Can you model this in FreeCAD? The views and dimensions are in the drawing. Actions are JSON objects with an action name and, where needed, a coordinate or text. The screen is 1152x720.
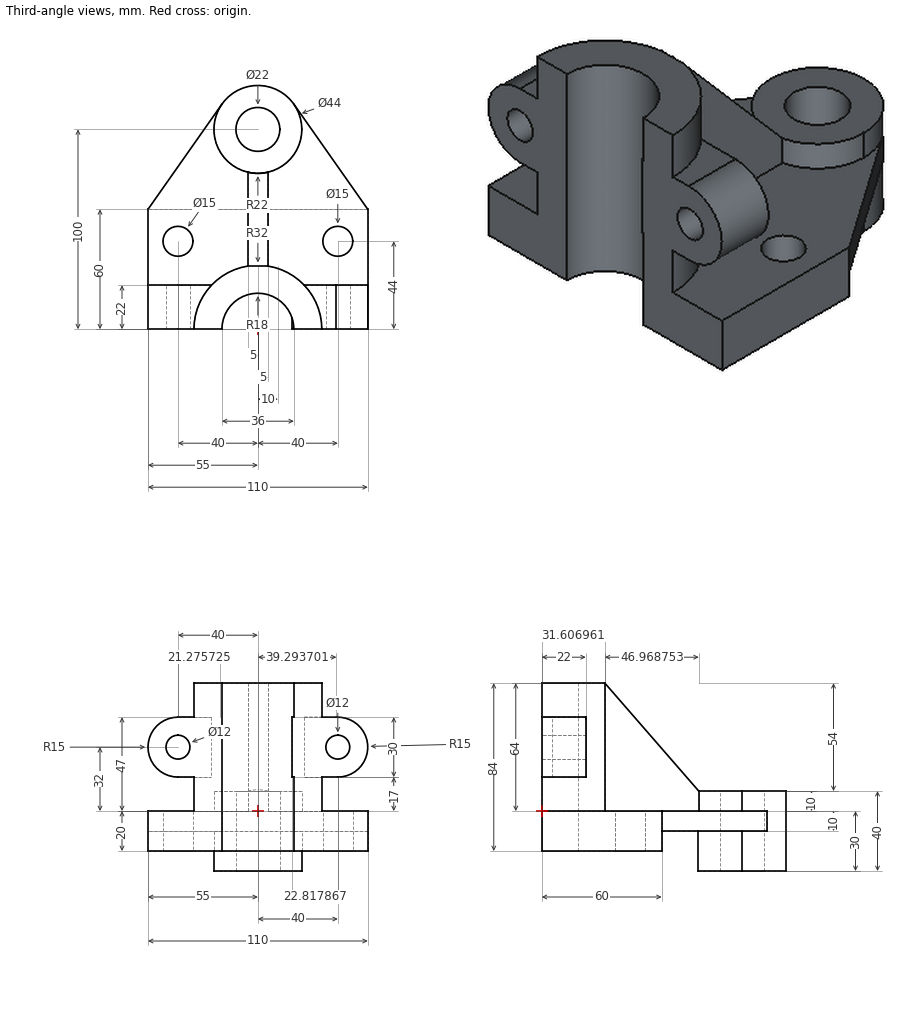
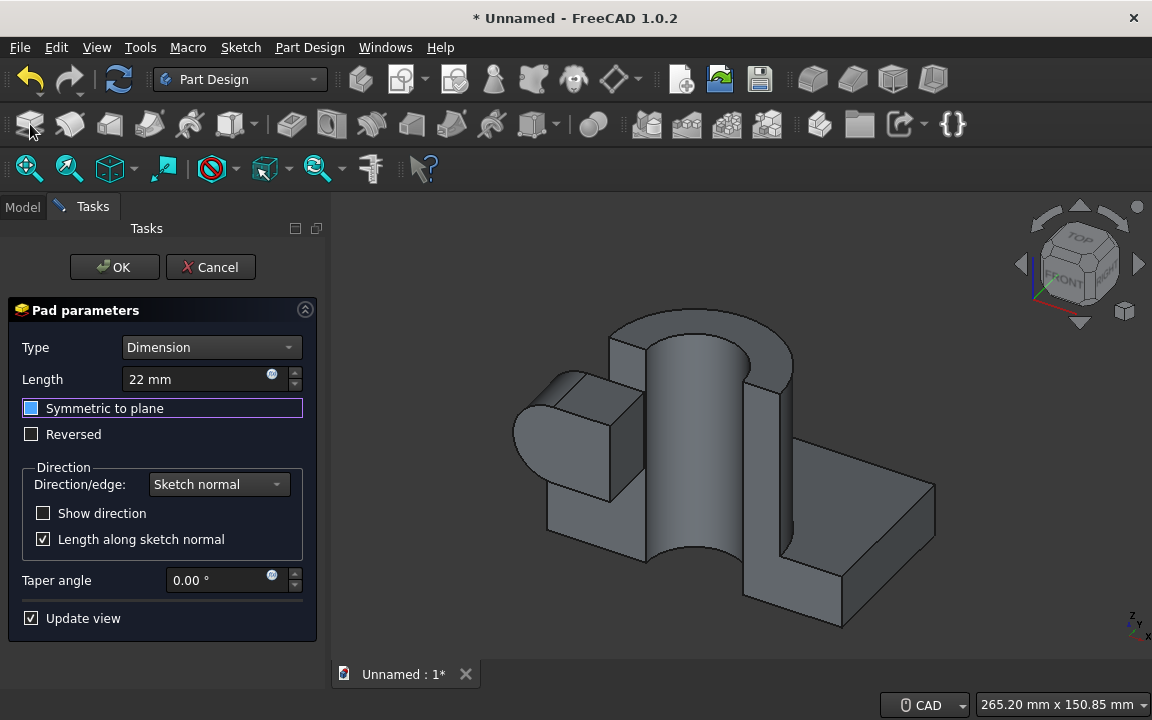
{"action": "left_click", "coordinate": [30, 434]}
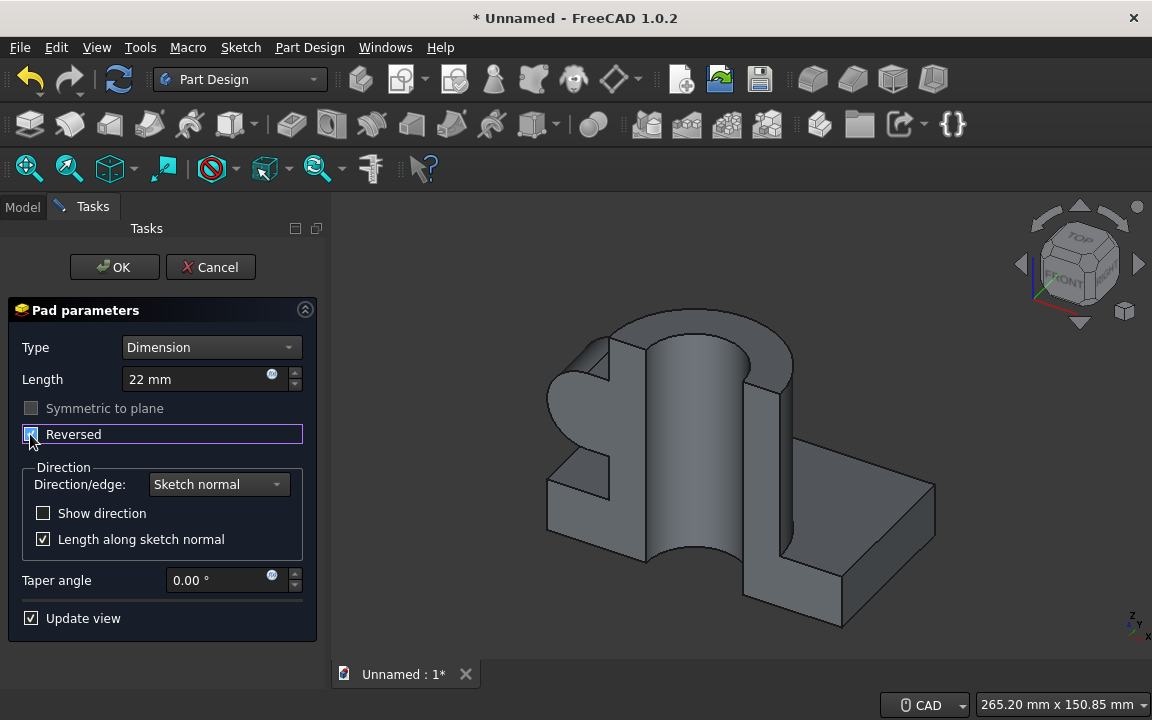
{"action": "left_click", "coordinate": [115, 267]}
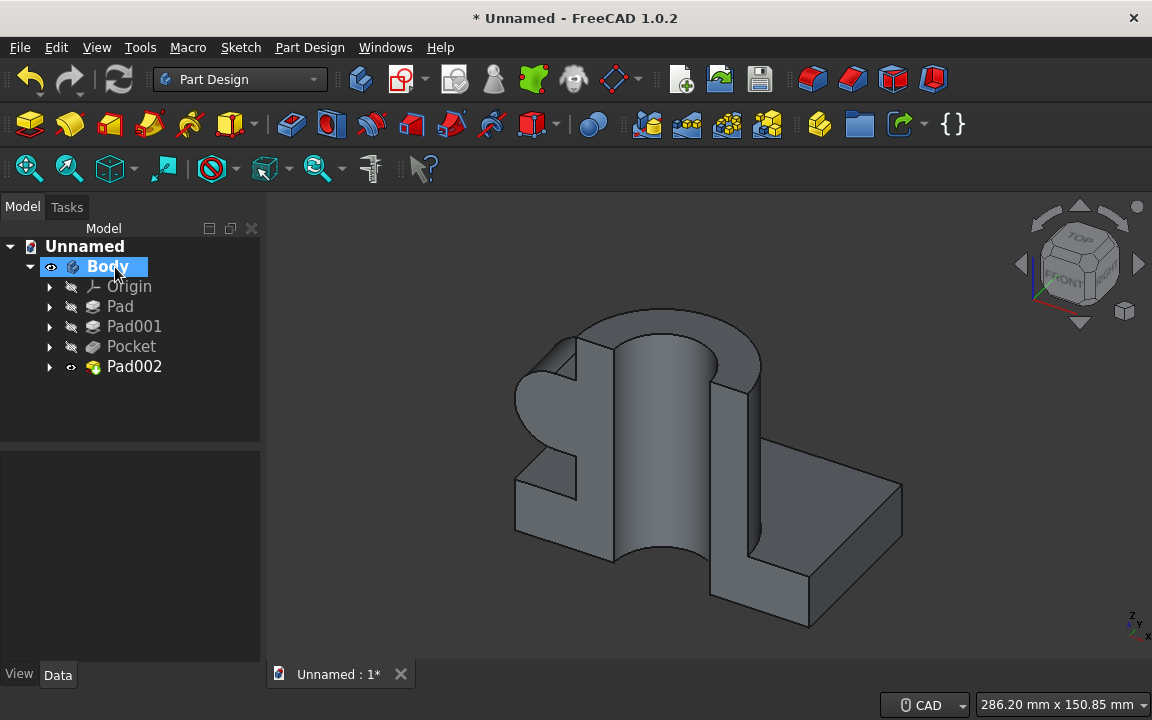
{"action": "key", "text": "4"}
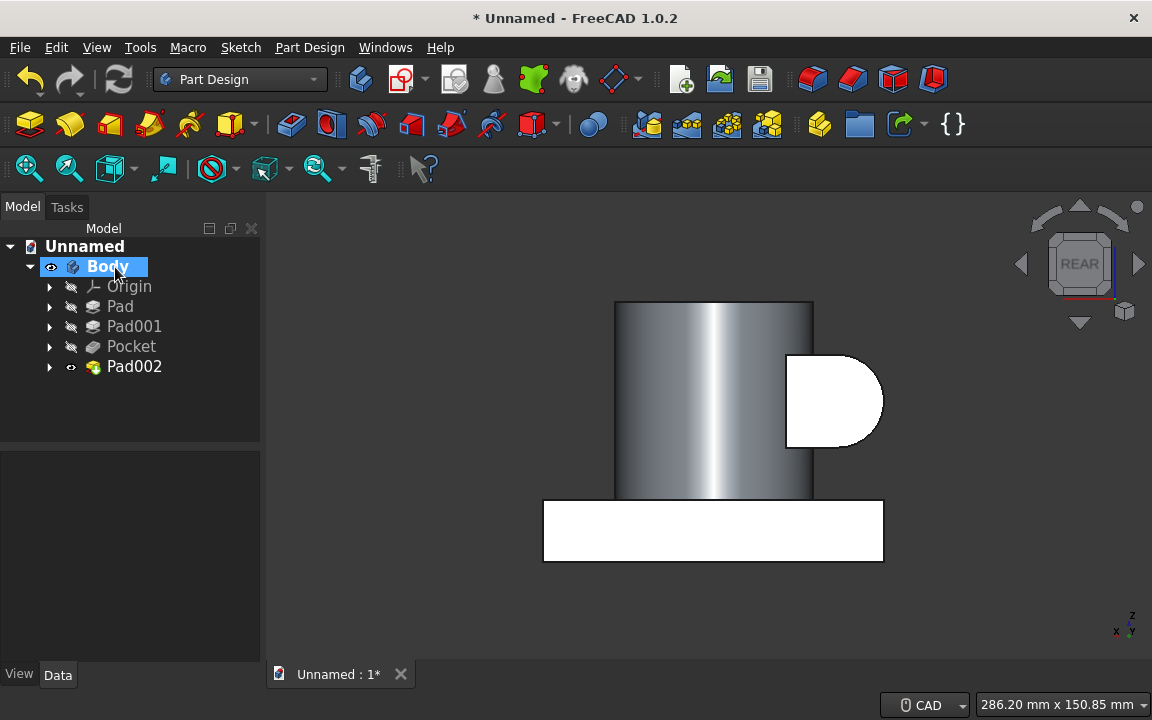
{"action": "left_click", "coordinate": [835, 400]}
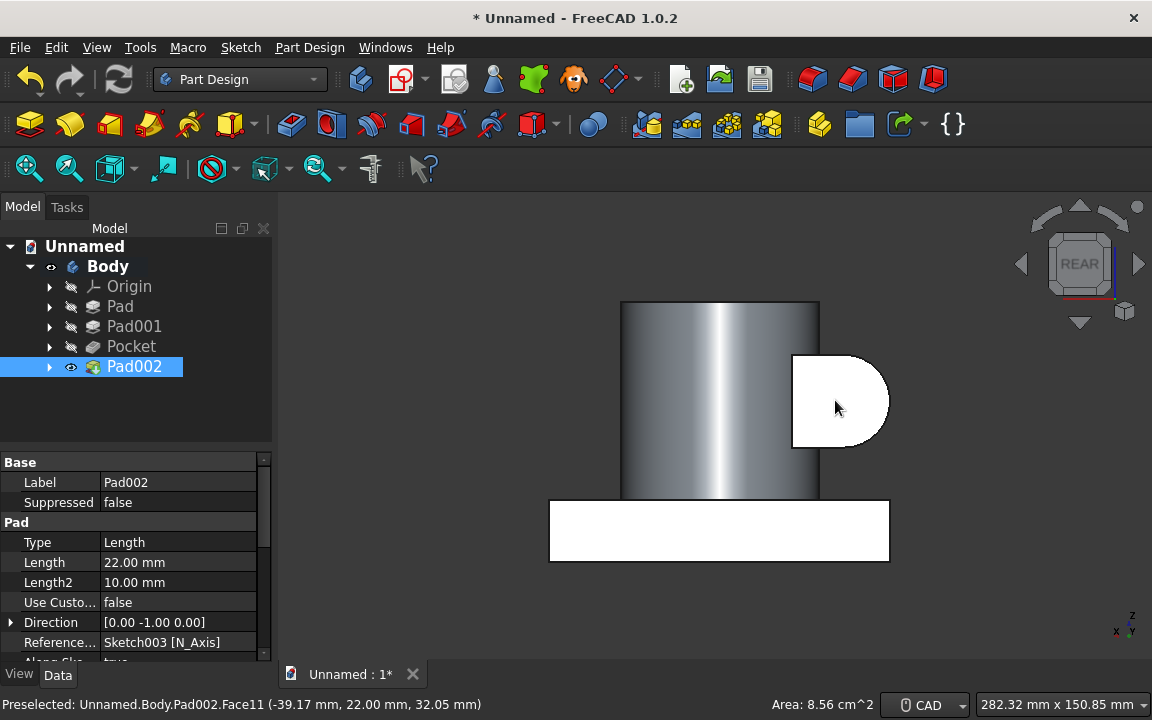
{"action": "left_click", "coordinate": [402, 80]}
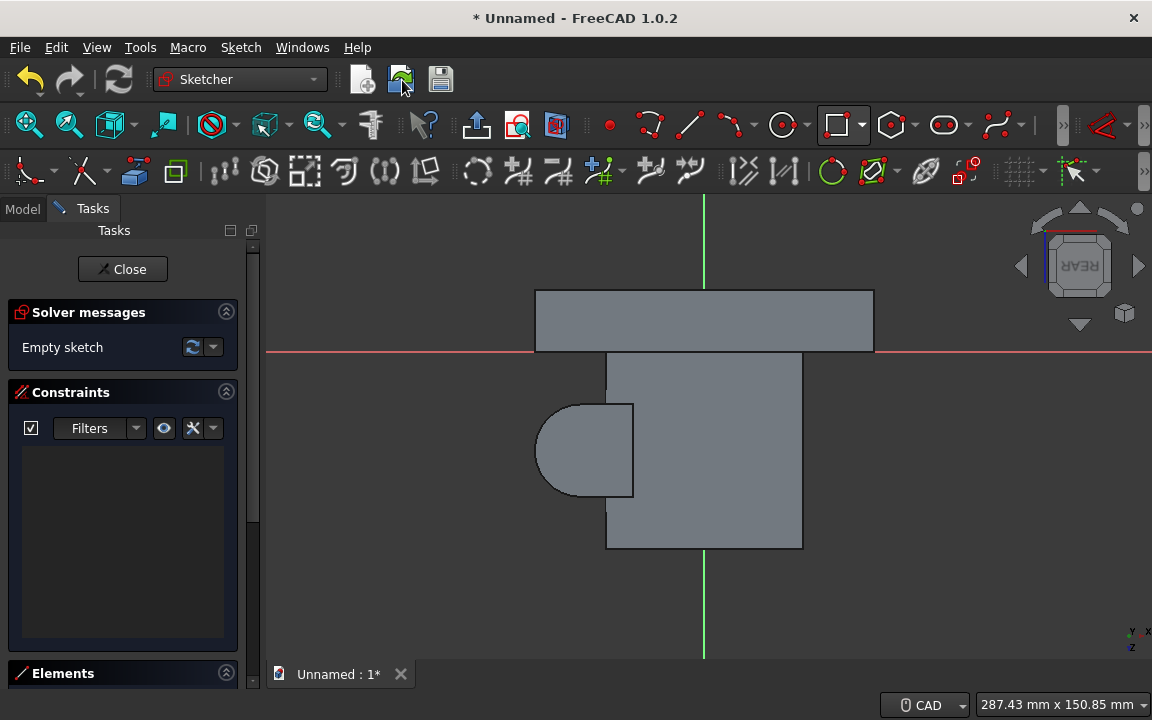
{"action": "left_click", "coordinate": [558, 126]}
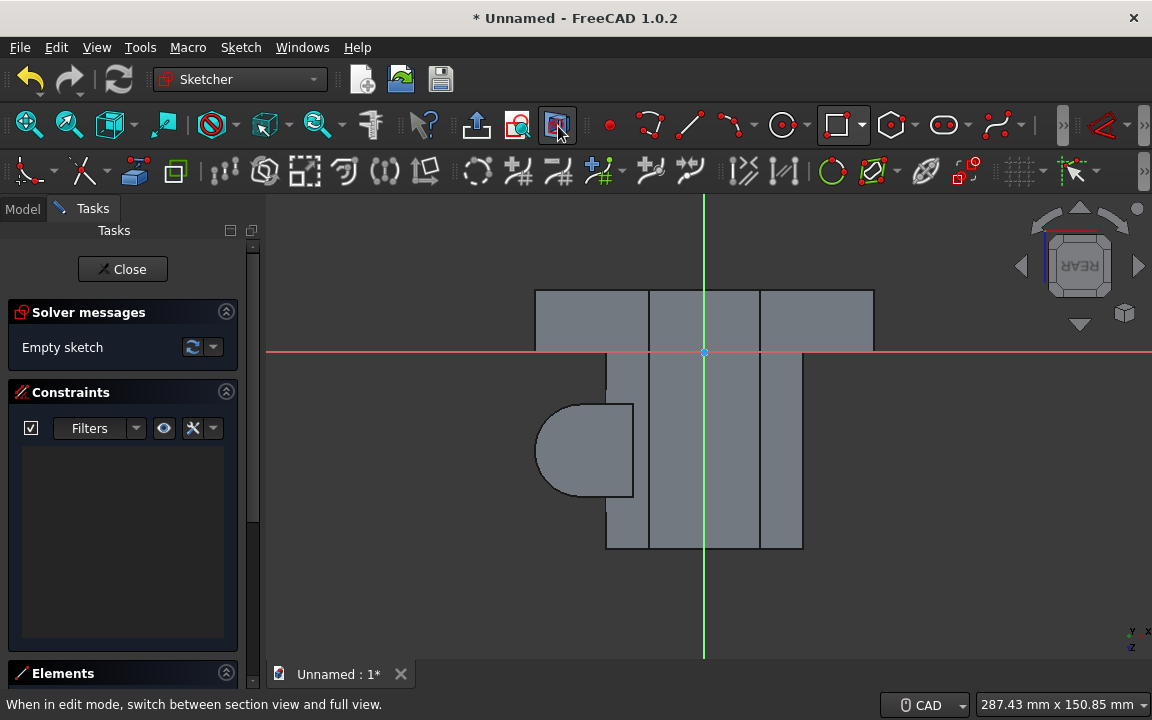
{"action": "scroll", "coordinate": [572, 455], "scroll_direction": "up", "scroll_amount": 10}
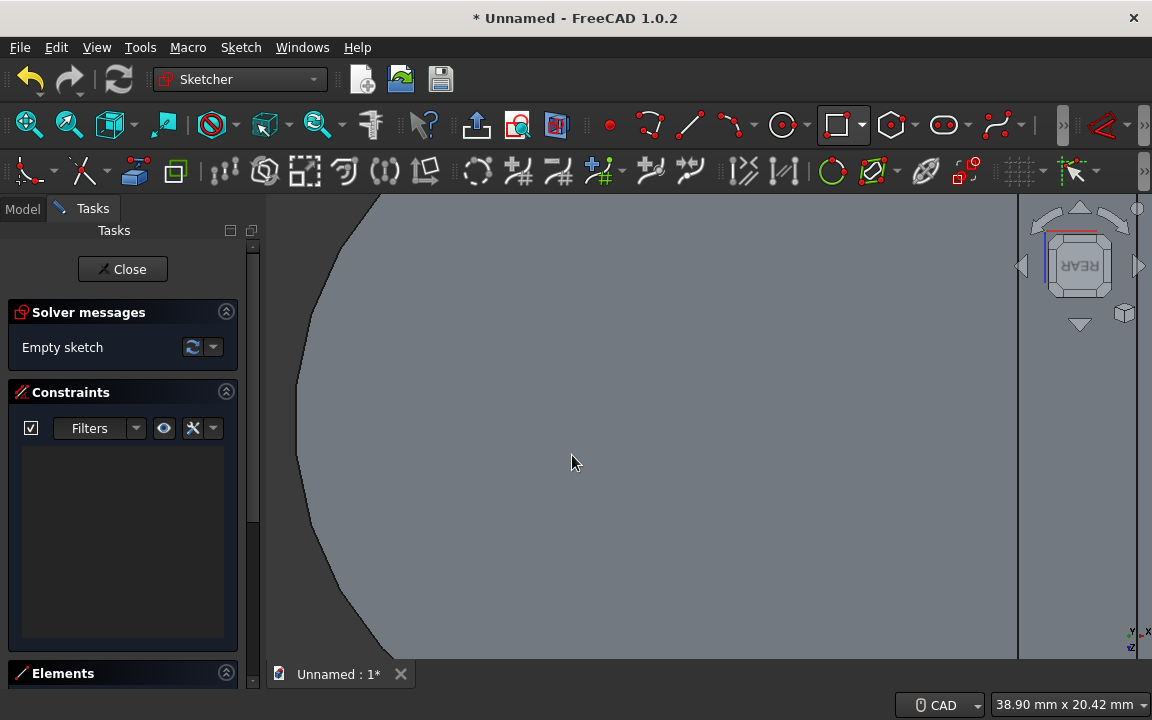
{"action": "left_click", "coordinate": [784, 126]}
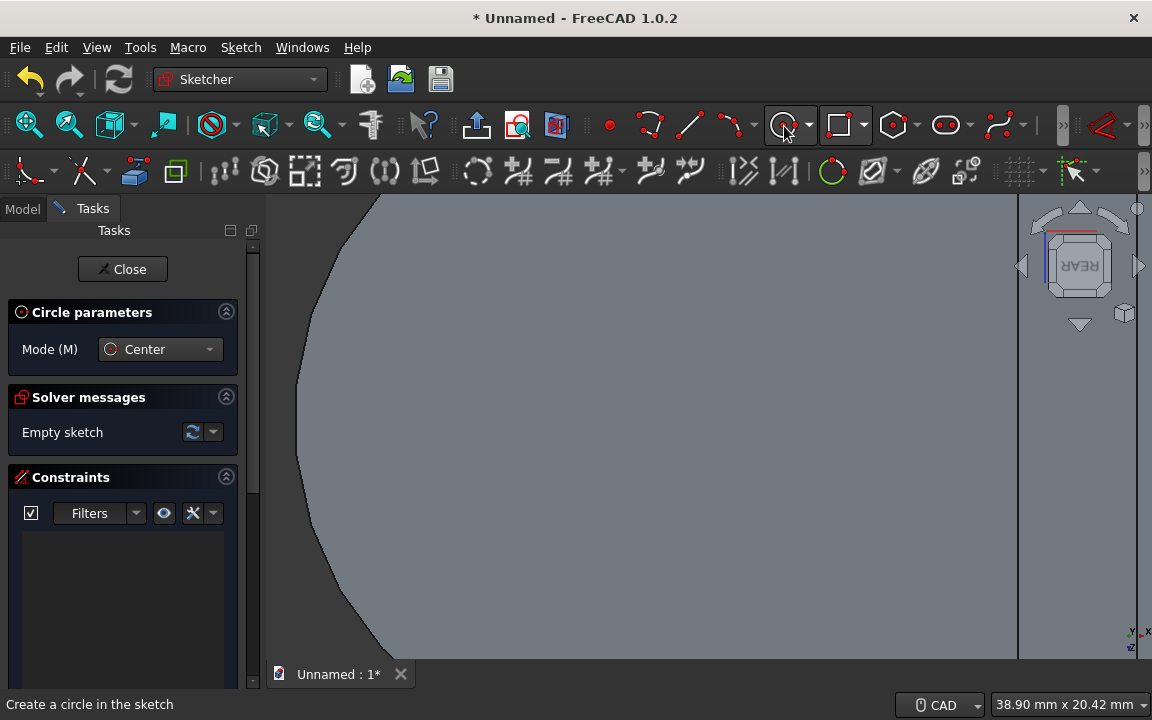
{"action": "left_click", "coordinate": [636, 420]}
{"action": "left_click", "coordinate": [733, 323]}
{"action": "key", "text": "Escape"}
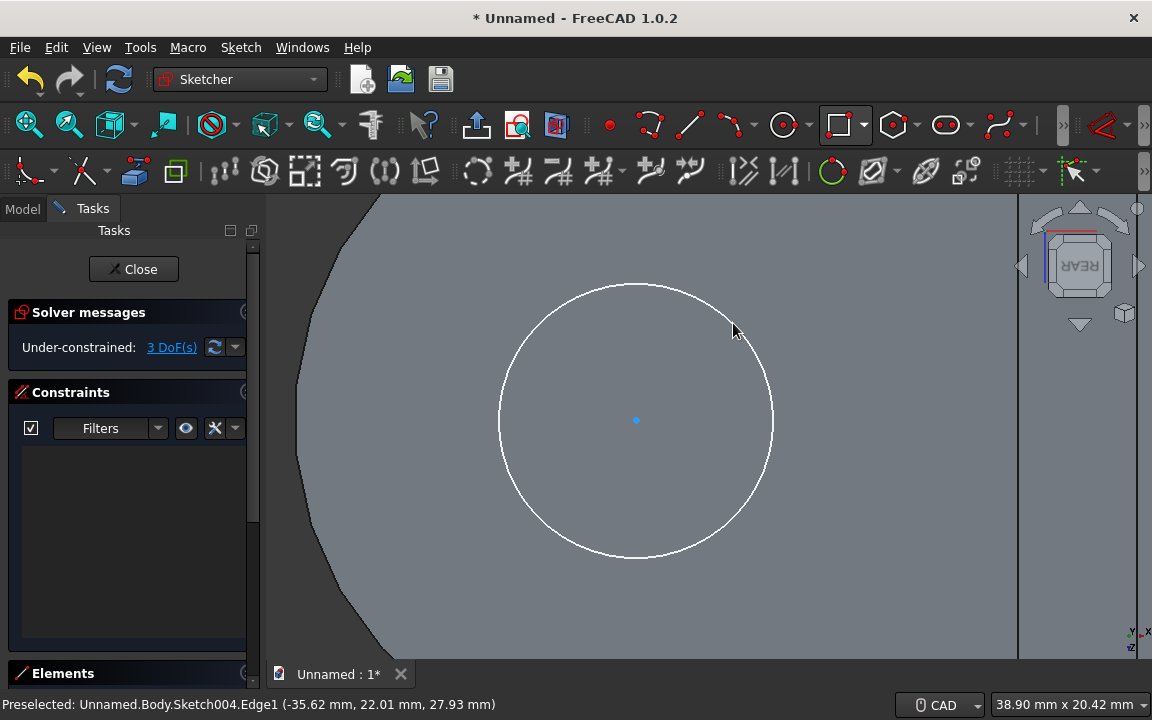
{"action": "left_click", "coordinate": [1102, 126]}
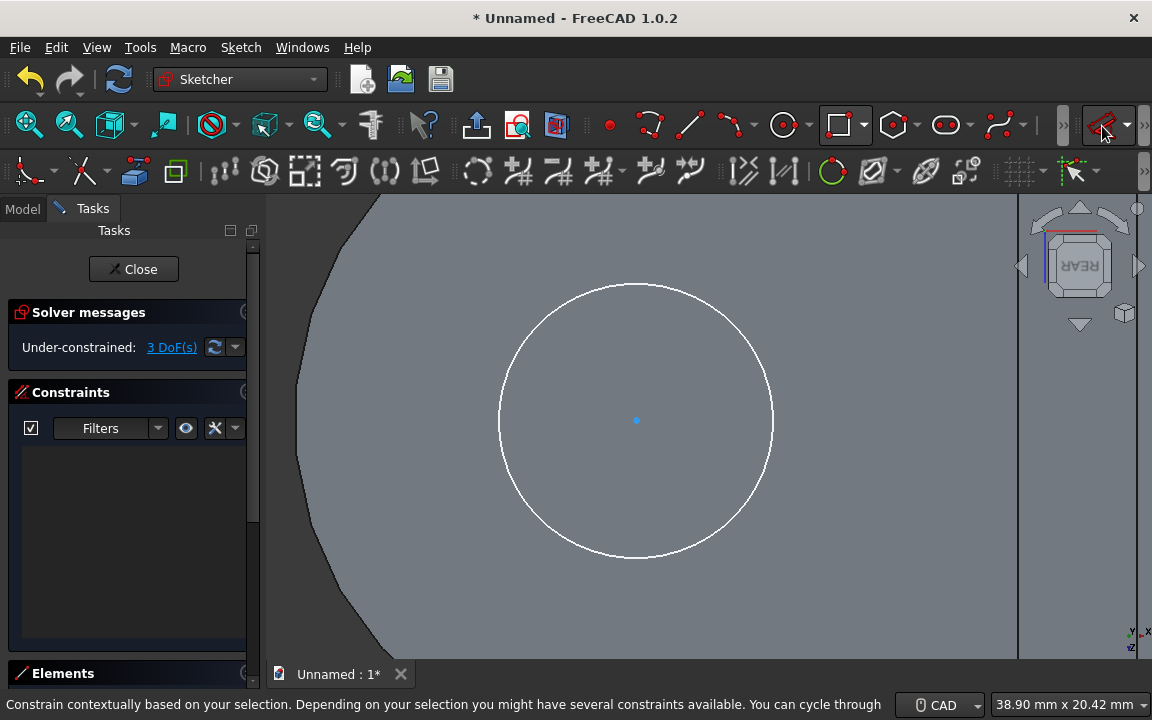
{"action": "left_click", "coordinate": [733, 324]}
{"action": "left_click", "coordinate": [756, 301]}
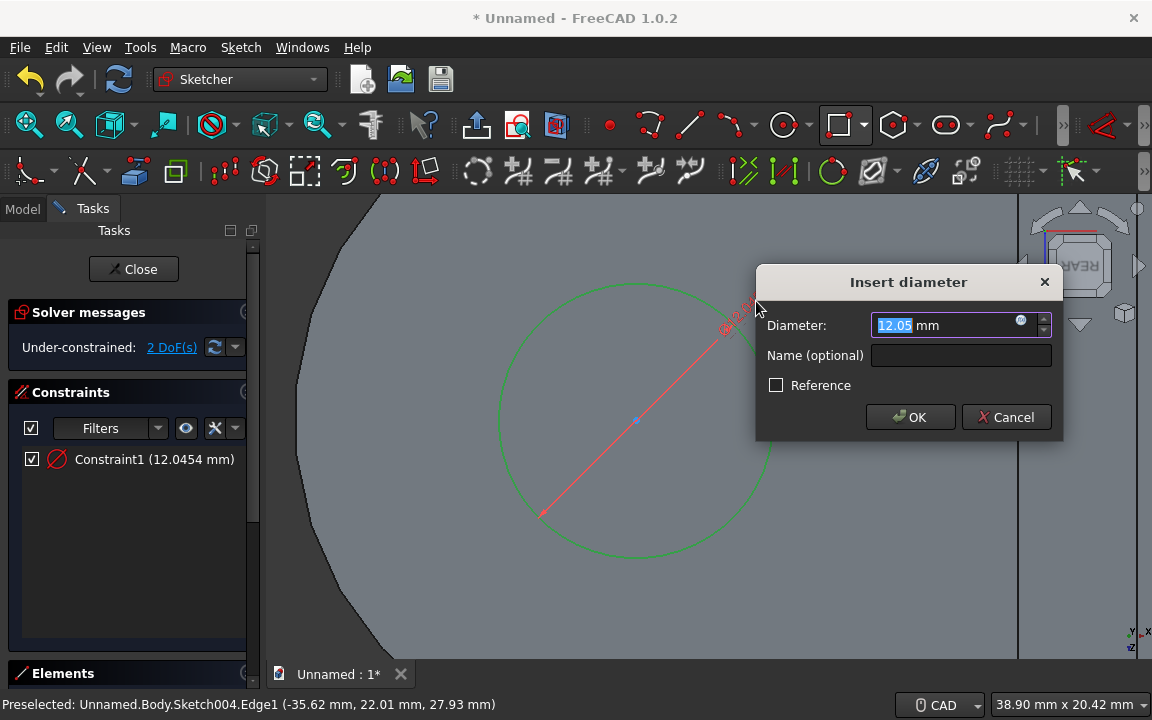
{"action": "type", "text": "12"}
{"action": "key", "text": "Return"}